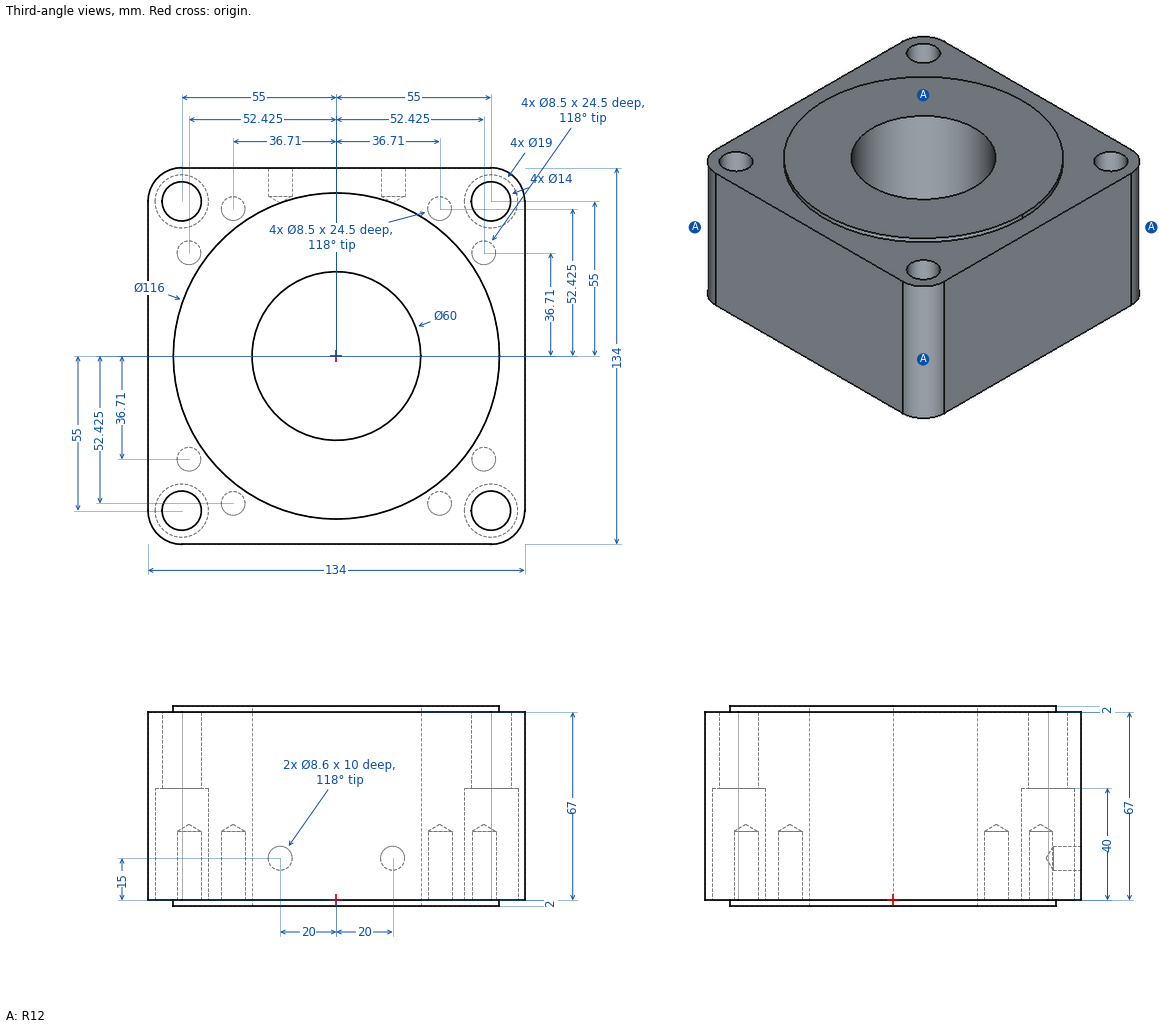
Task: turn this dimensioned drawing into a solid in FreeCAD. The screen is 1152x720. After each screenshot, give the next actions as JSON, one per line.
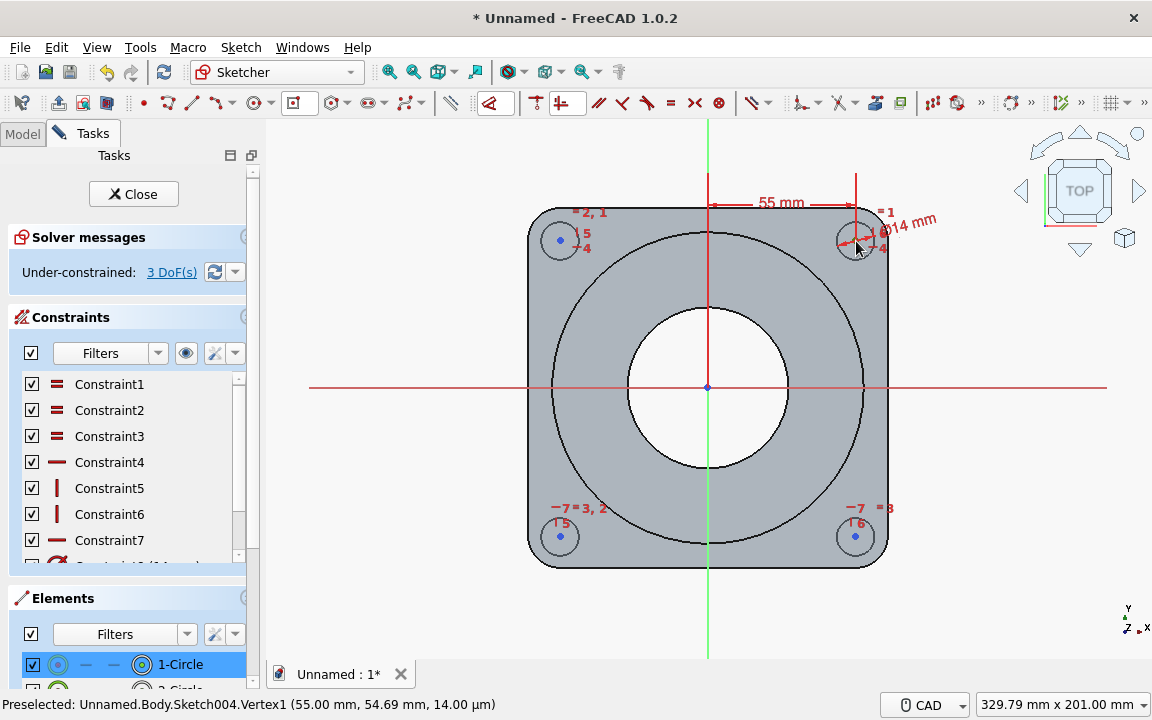
{"action": "key", "text": "i"}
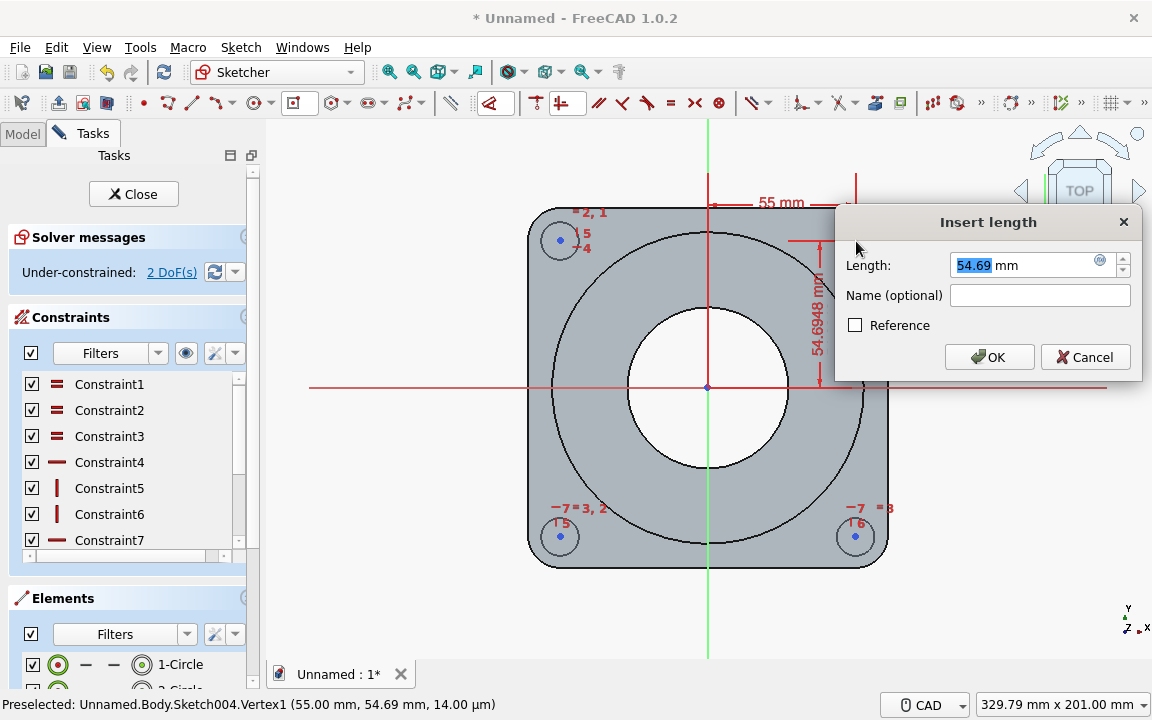
{"action": "type", "text": "55"}
{"action": "key", "text": "Return"}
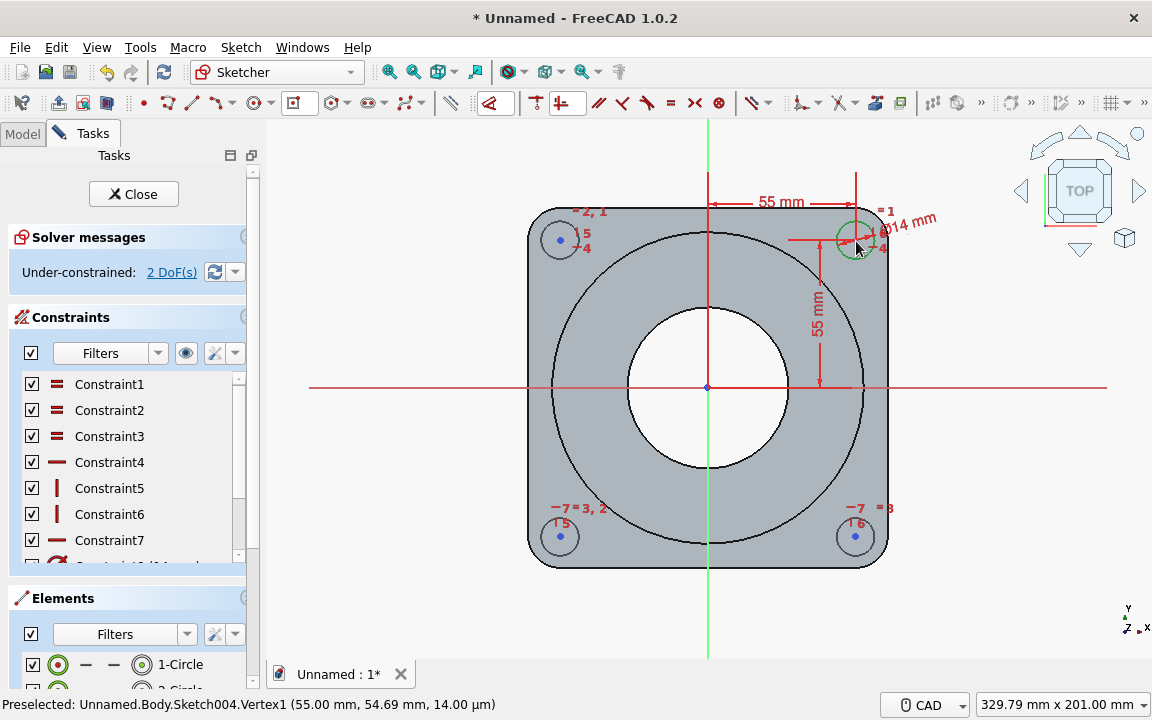
{"action": "left_click", "coordinate": [560, 240]}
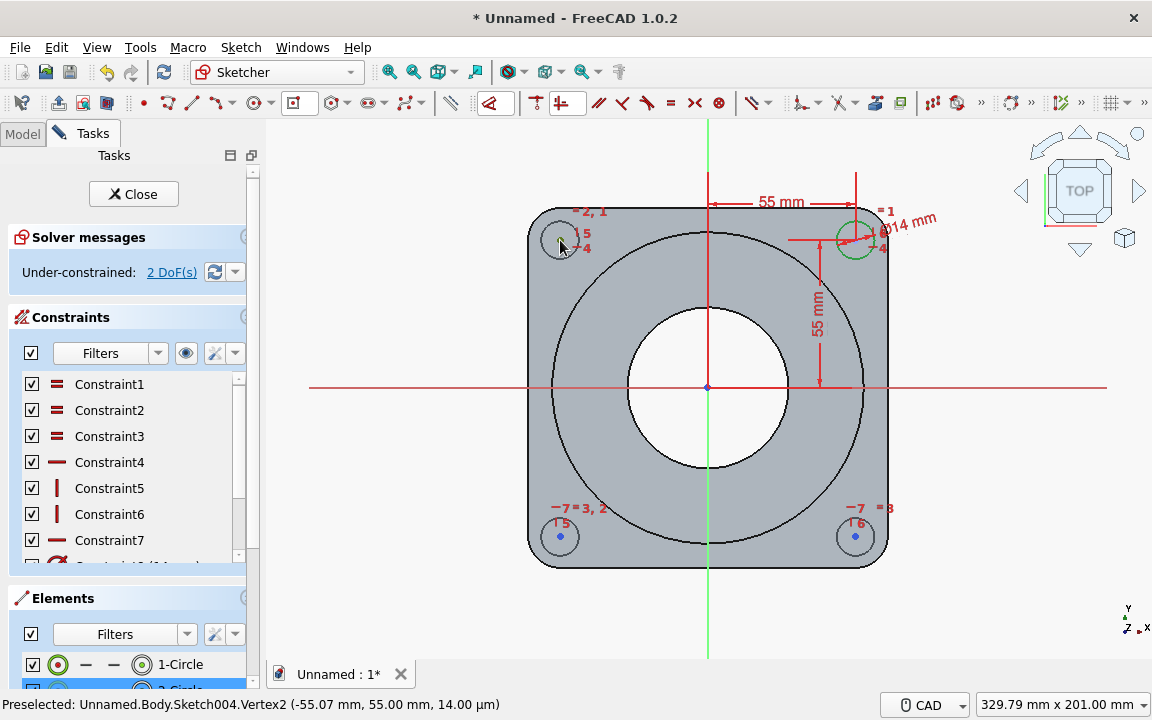
{"action": "left_click", "coordinate": [508, 104]}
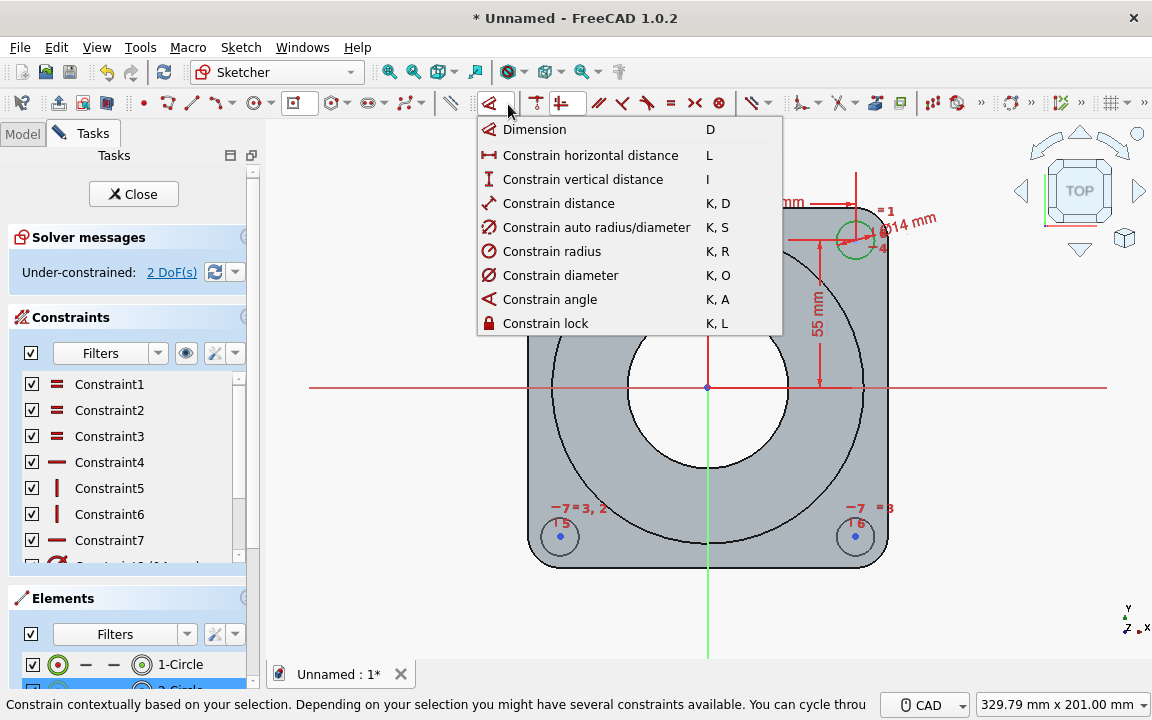
{"action": "left_click", "coordinate": [630, 155]}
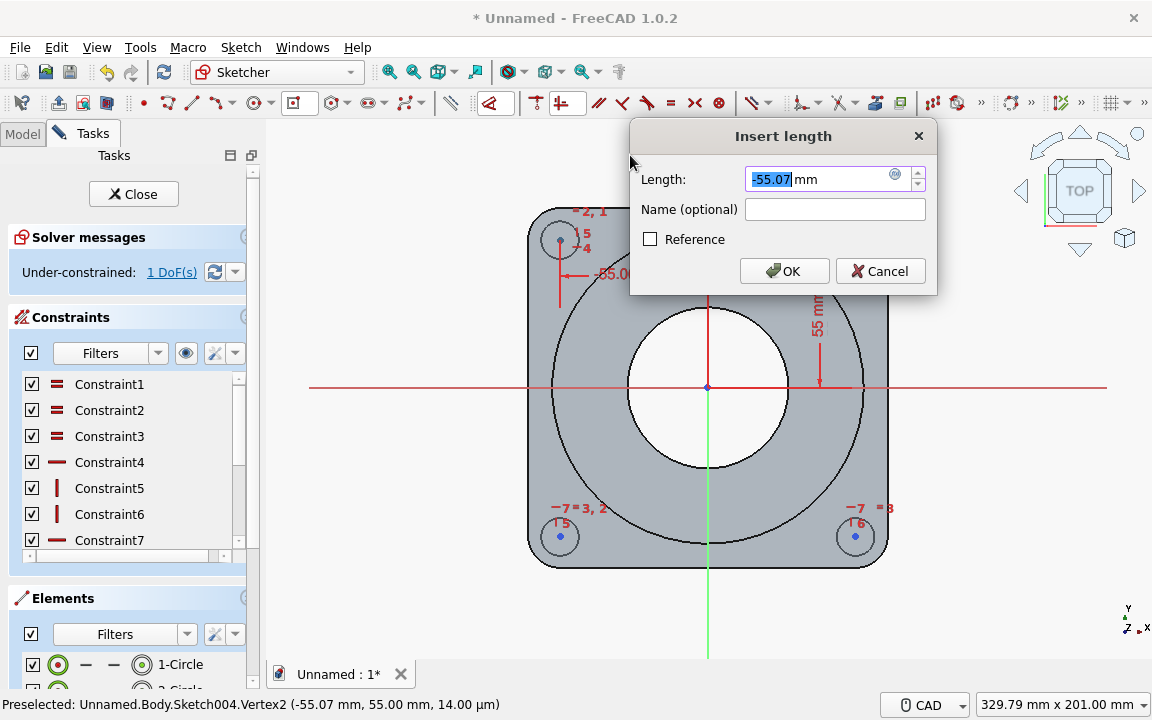
{"action": "type", "text": "-55"}
{"action": "key", "text": "Return"}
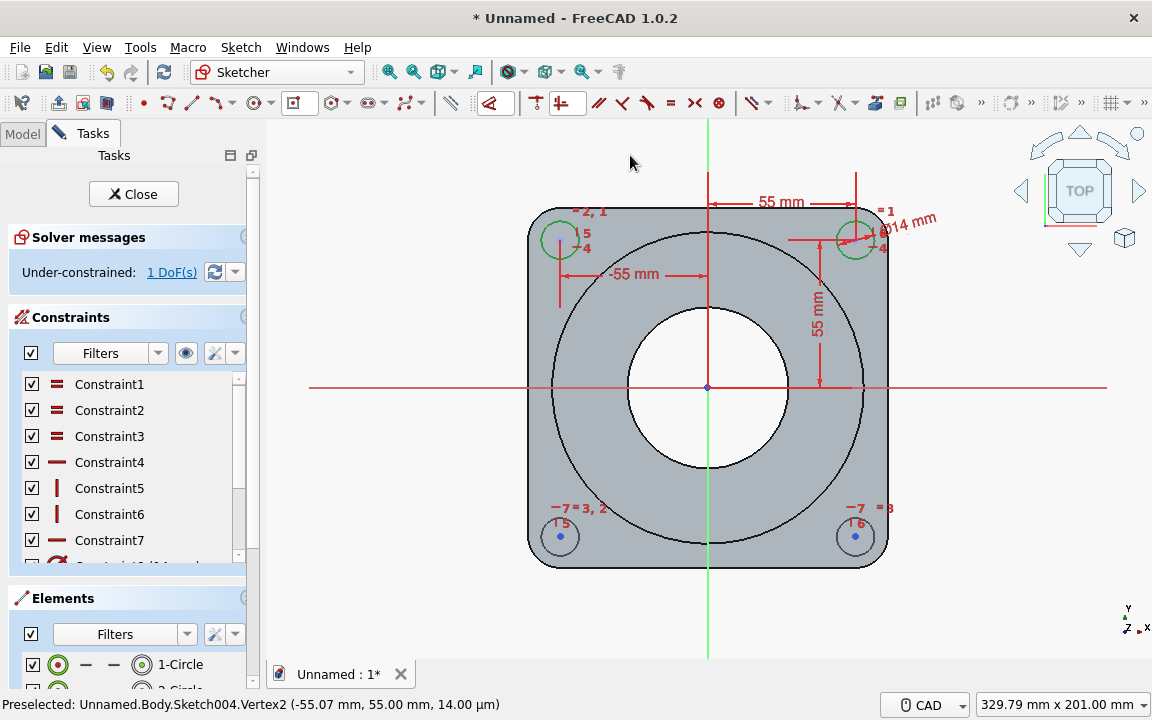
{"action": "left_click", "coordinate": [560, 537]}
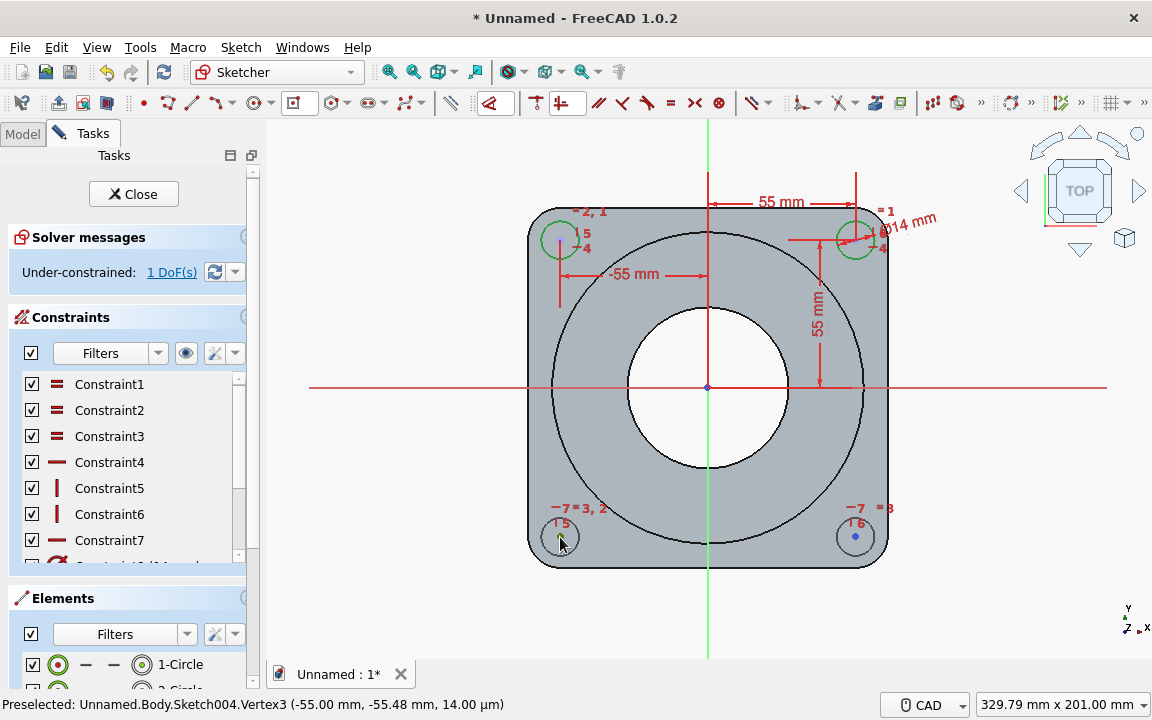
{"action": "left_click", "coordinate": [508, 104]}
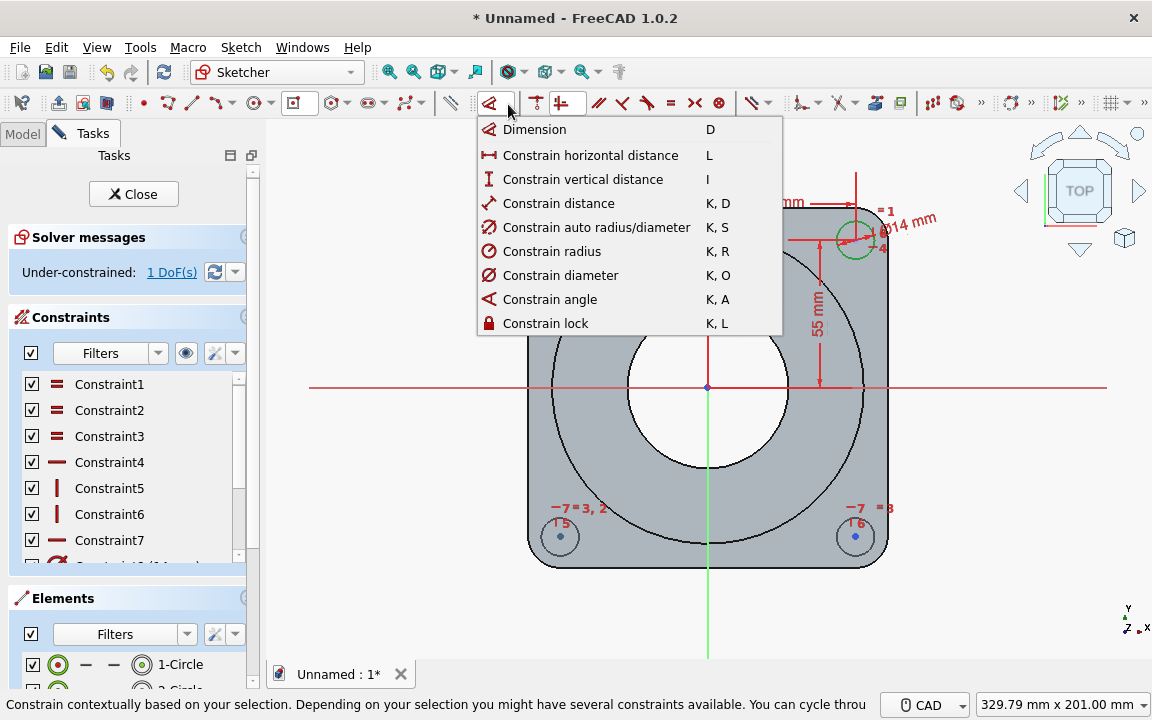
{"action": "left_click", "coordinate": [630, 179]}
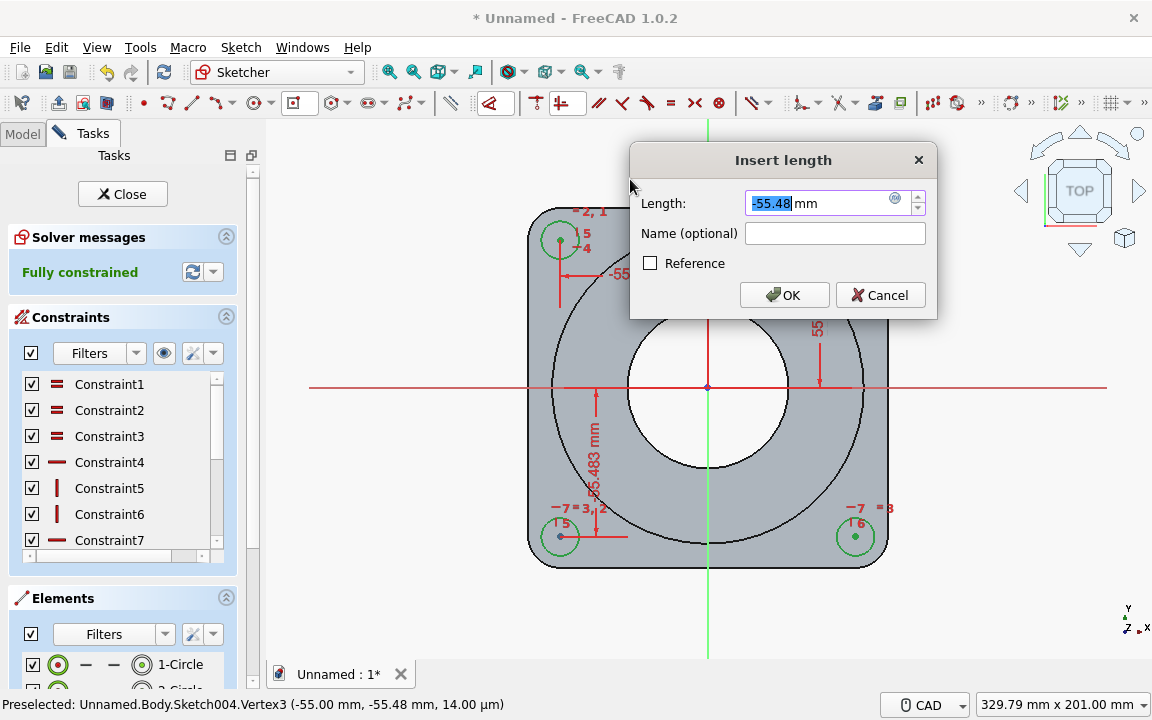
{"action": "type", "text": "-55"}
{"action": "key", "text": "Return"}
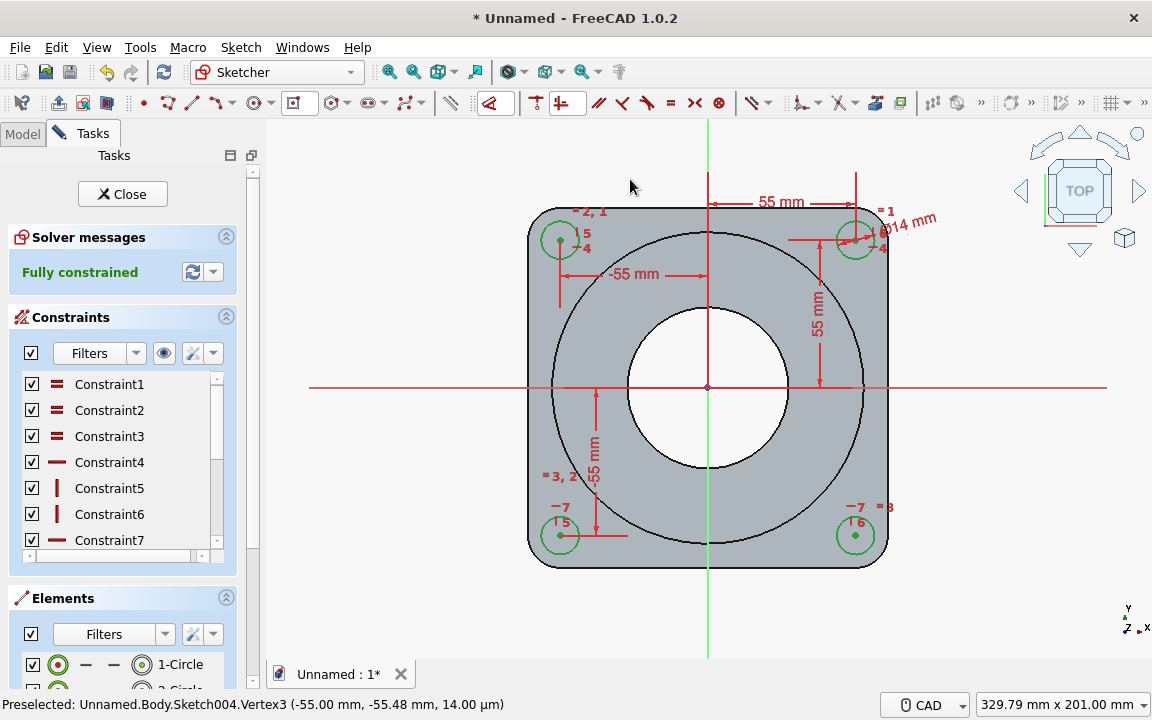
{"action": "left_click", "coordinate": [123, 194]}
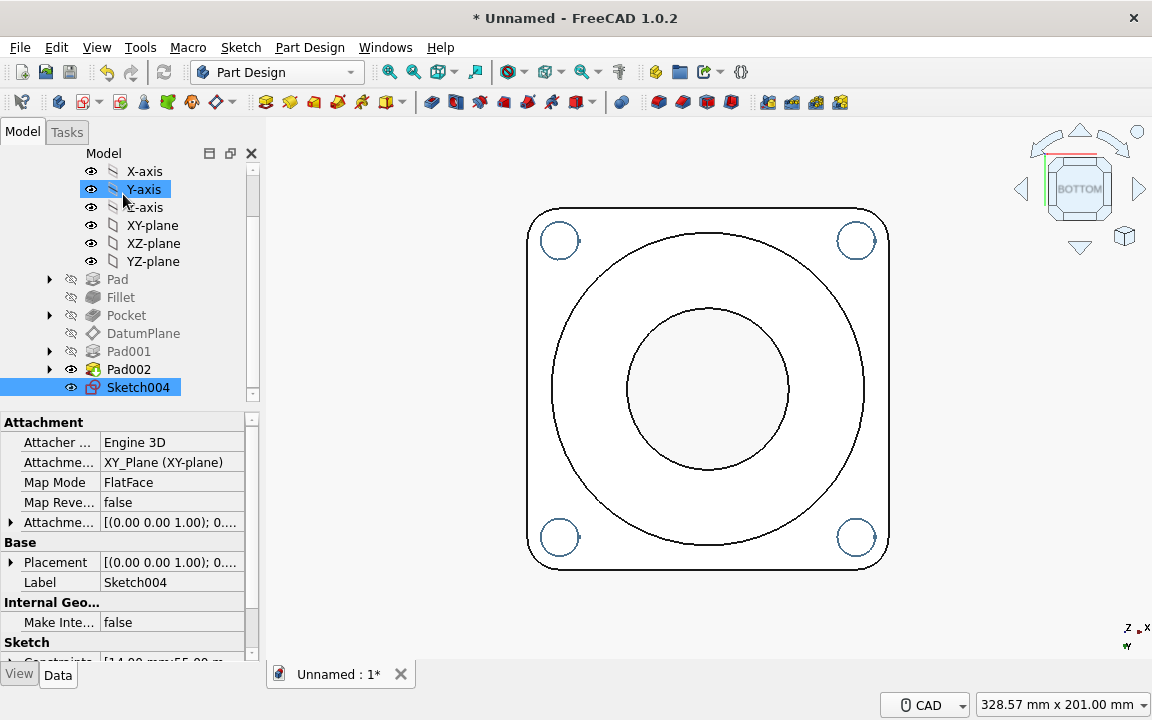
{"action": "left_click", "coordinate": [432, 102]}